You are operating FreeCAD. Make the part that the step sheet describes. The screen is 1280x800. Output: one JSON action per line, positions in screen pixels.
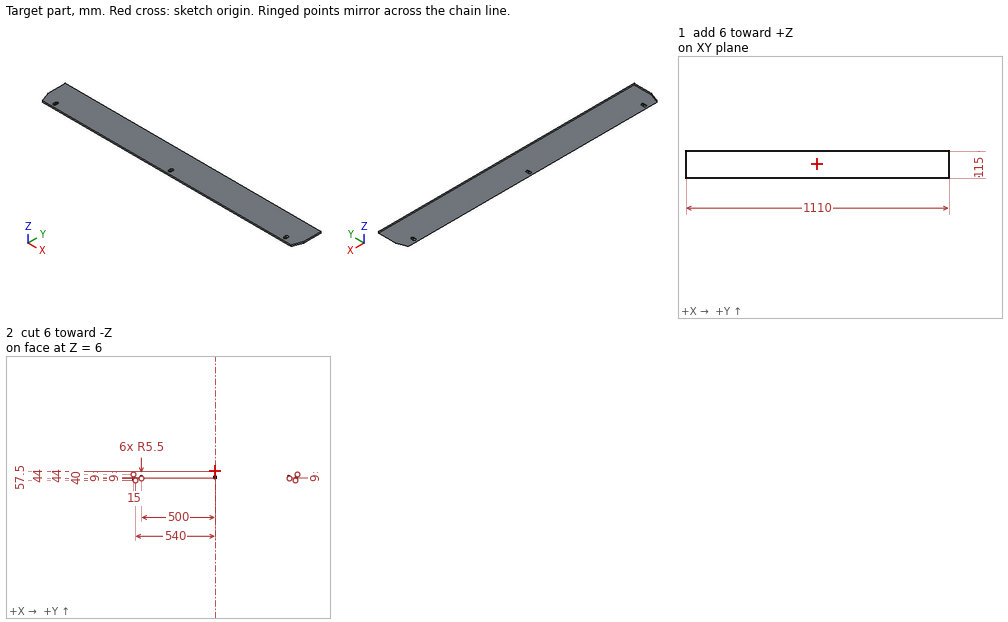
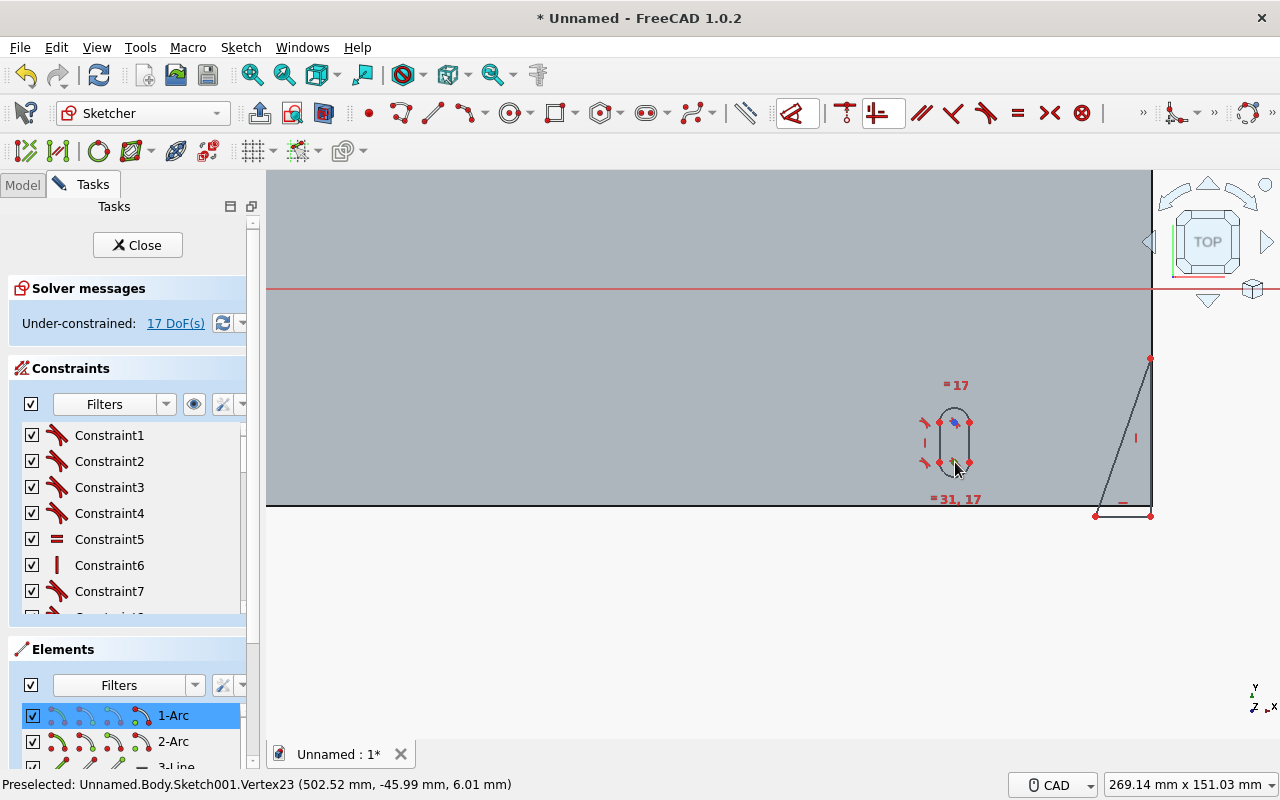
{"action": "scroll", "coordinate": [962, 463], "scroll_direction": "down", "scroll_amount": 10}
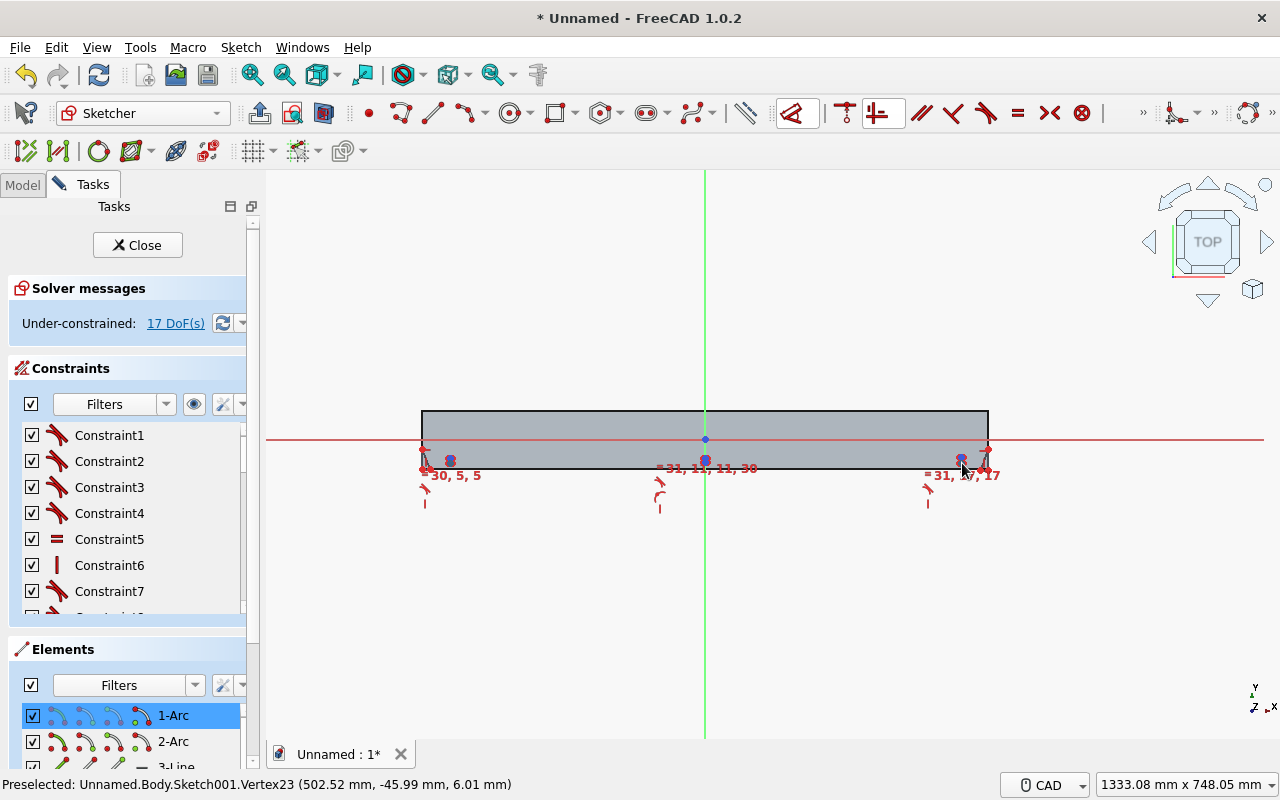
{"action": "left_click", "coordinate": [705, 674]}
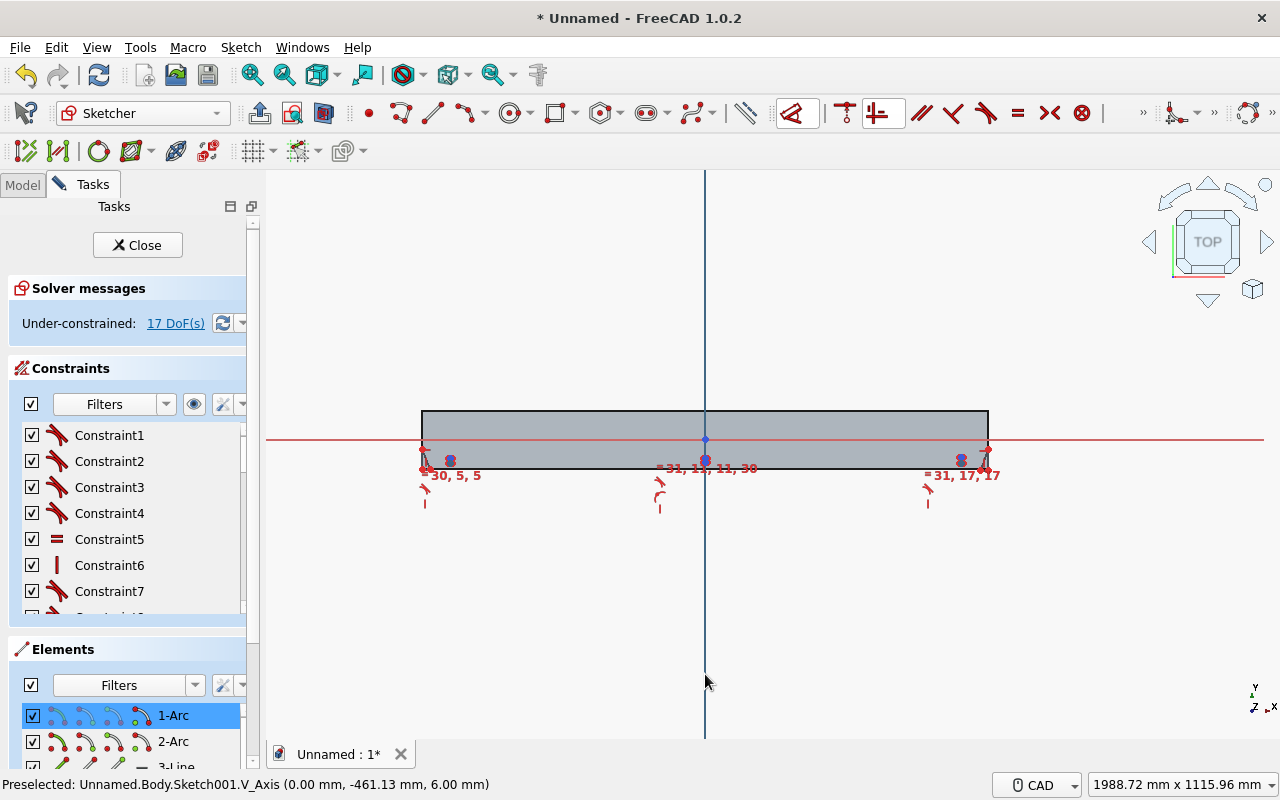
{"action": "left_click", "coordinate": [1050, 114]}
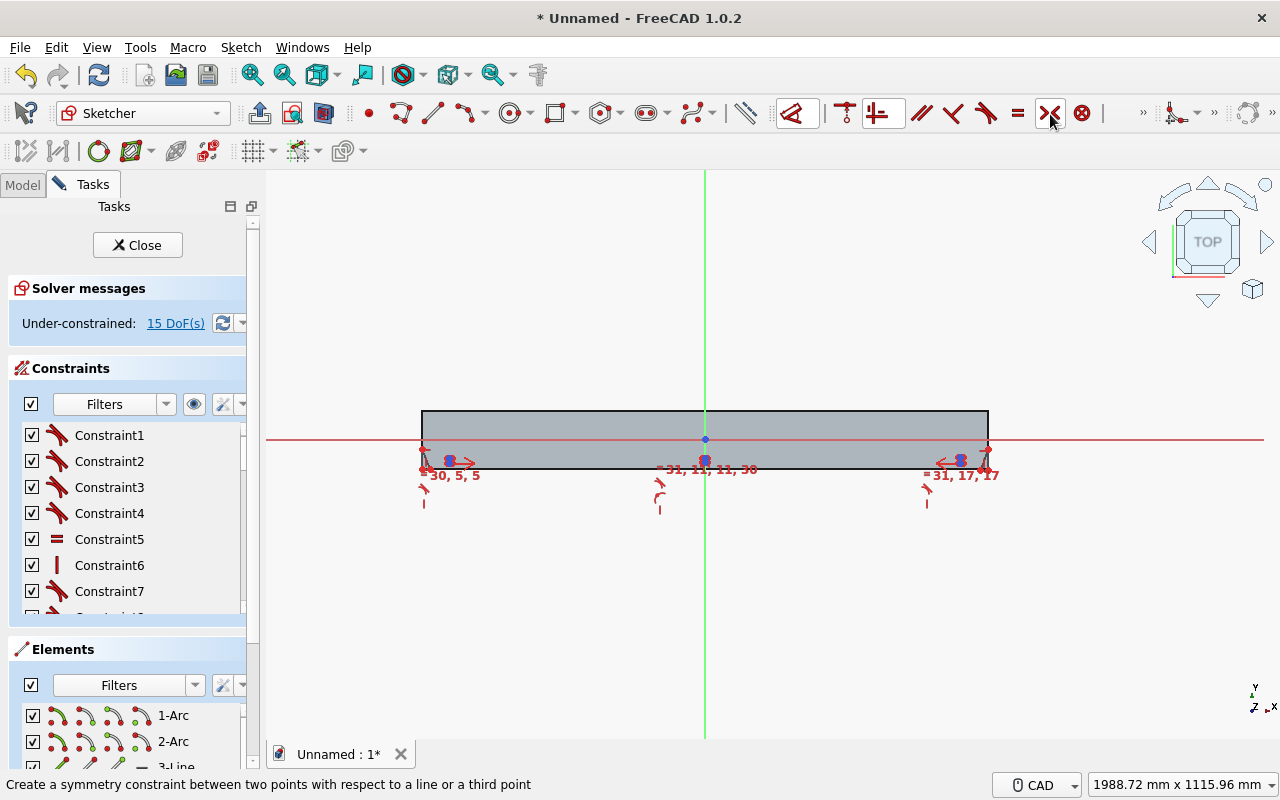
{"action": "scroll", "coordinate": [430, 470], "scroll_direction": "up", "scroll_amount": 3}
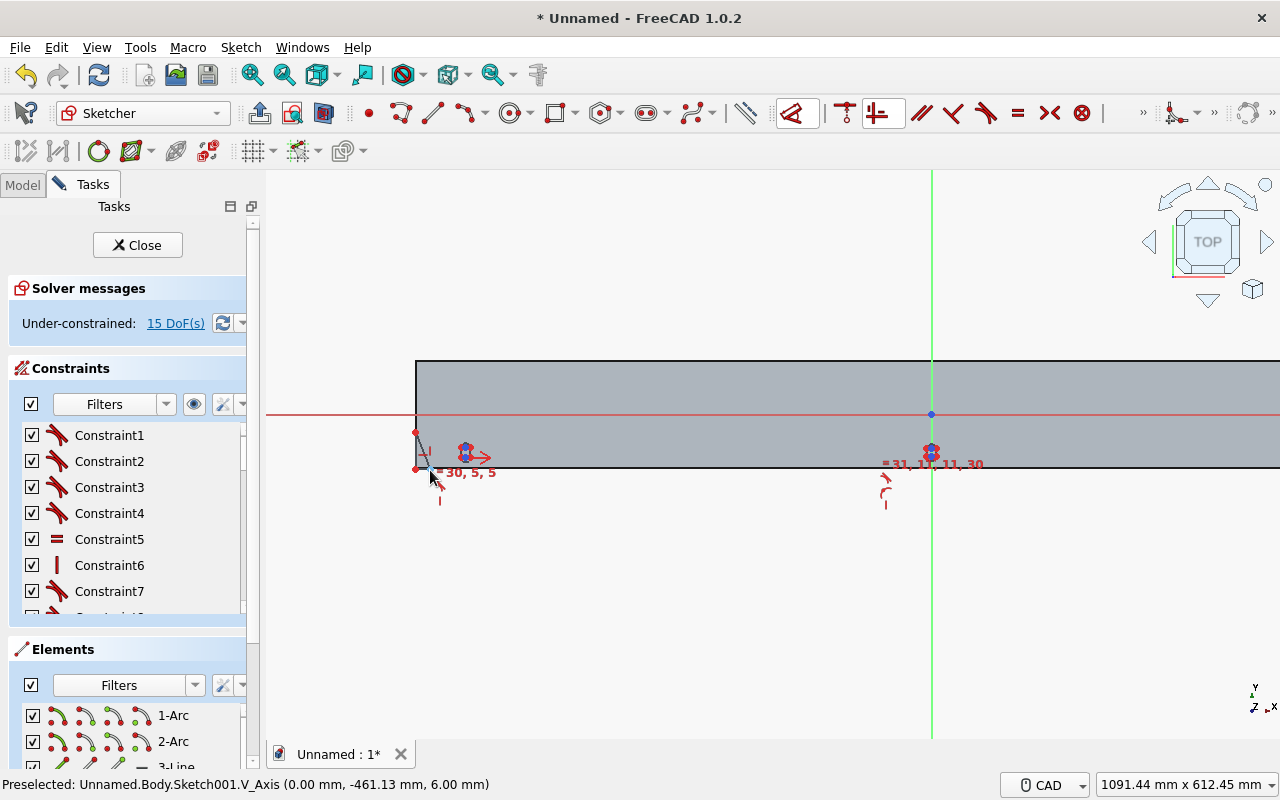
{"action": "left_click", "coordinate": [430, 469]}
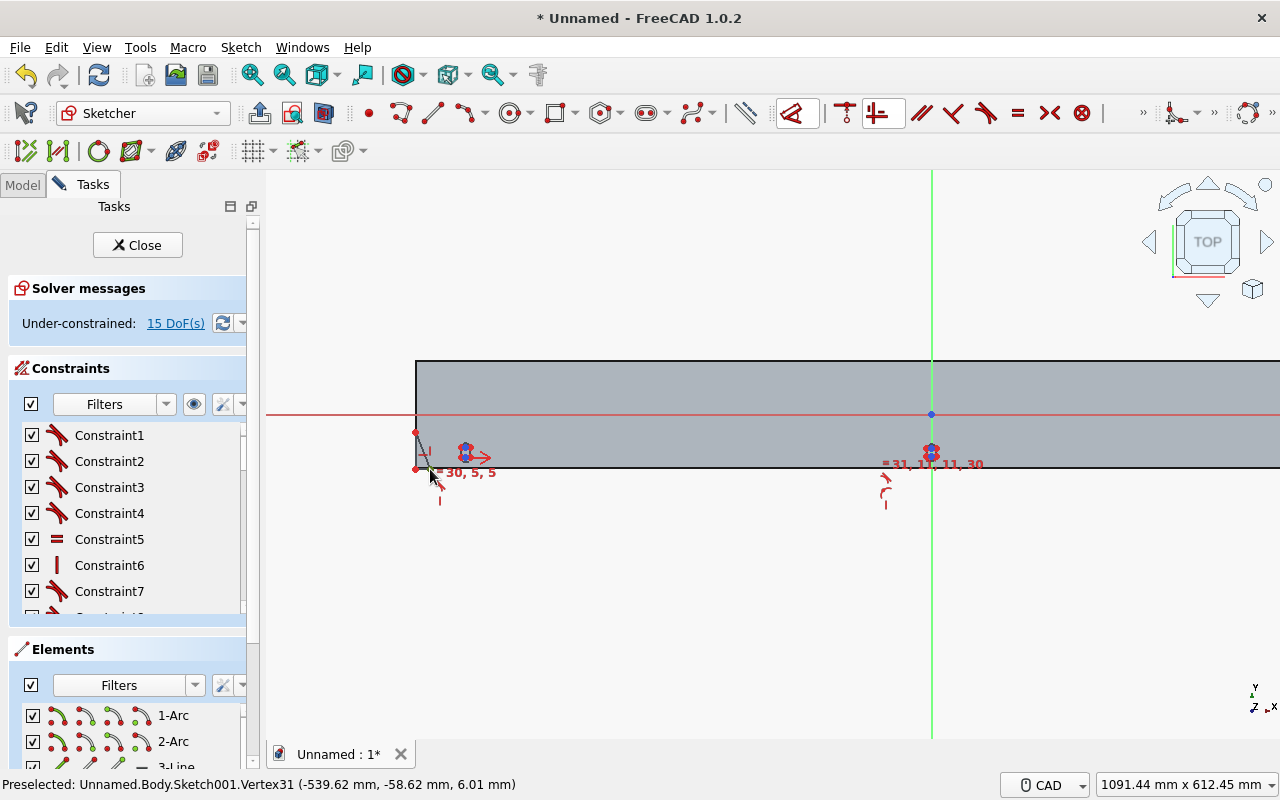
{"action": "scroll", "coordinate": [428, 470], "scroll_direction": "down", "scroll_amount": 3}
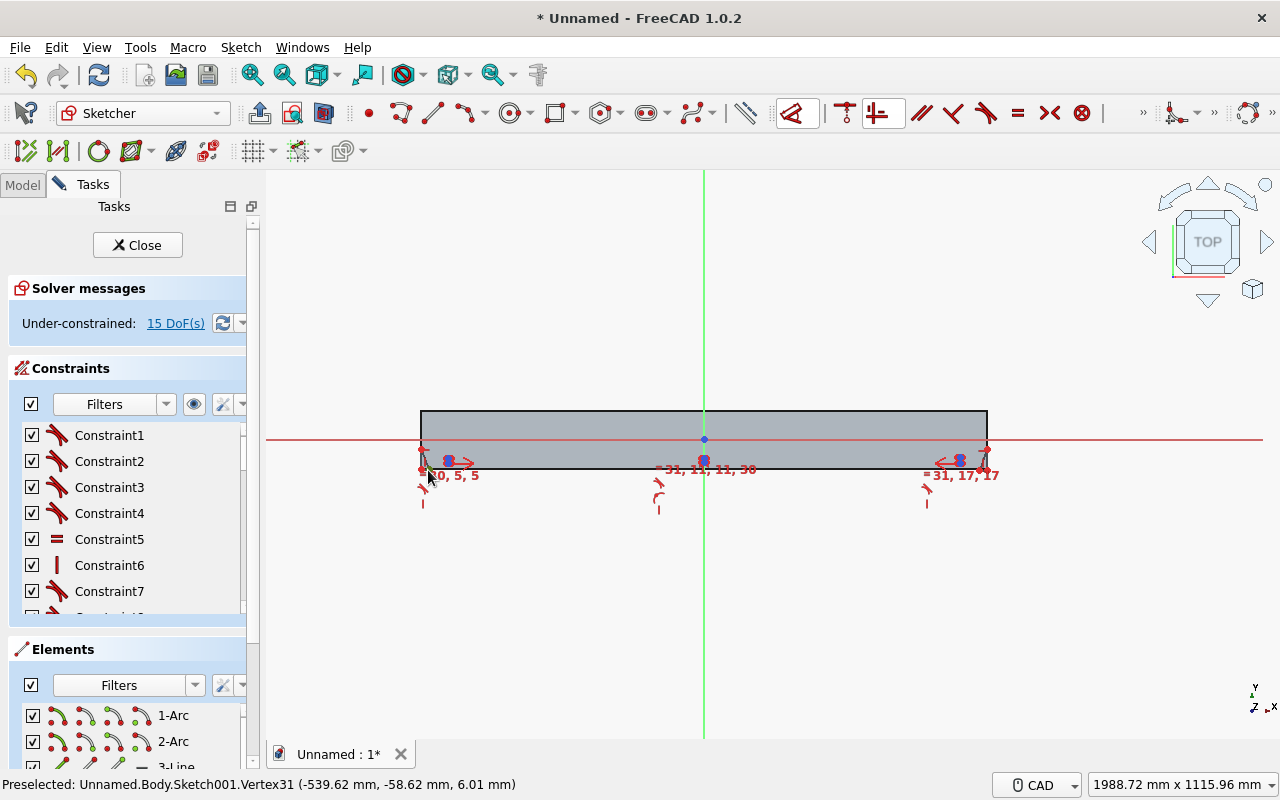
{"action": "scroll", "coordinate": [980, 471], "scroll_direction": "up", "scroll_amount": 3}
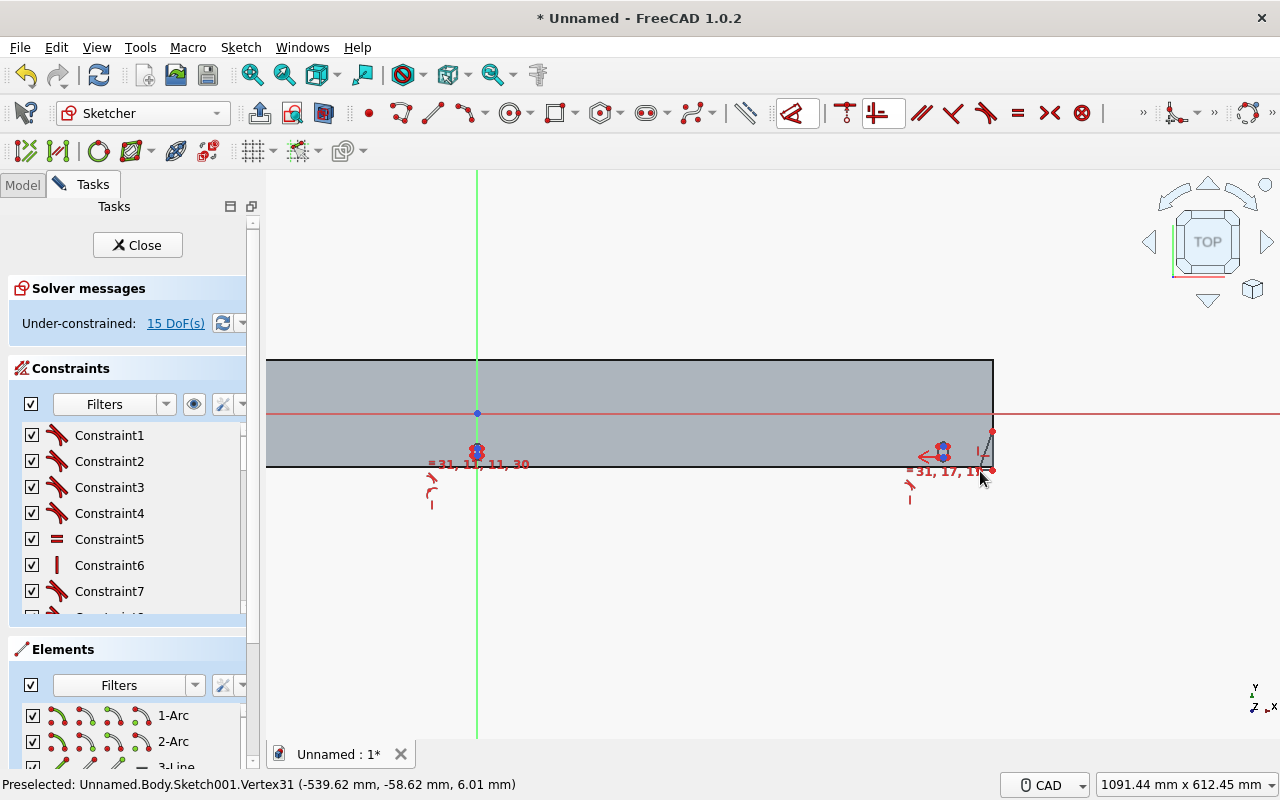
{"action": "scroll", "coordinate": [979, 470], "scroll_direction": "up", "scroll_amount": 4}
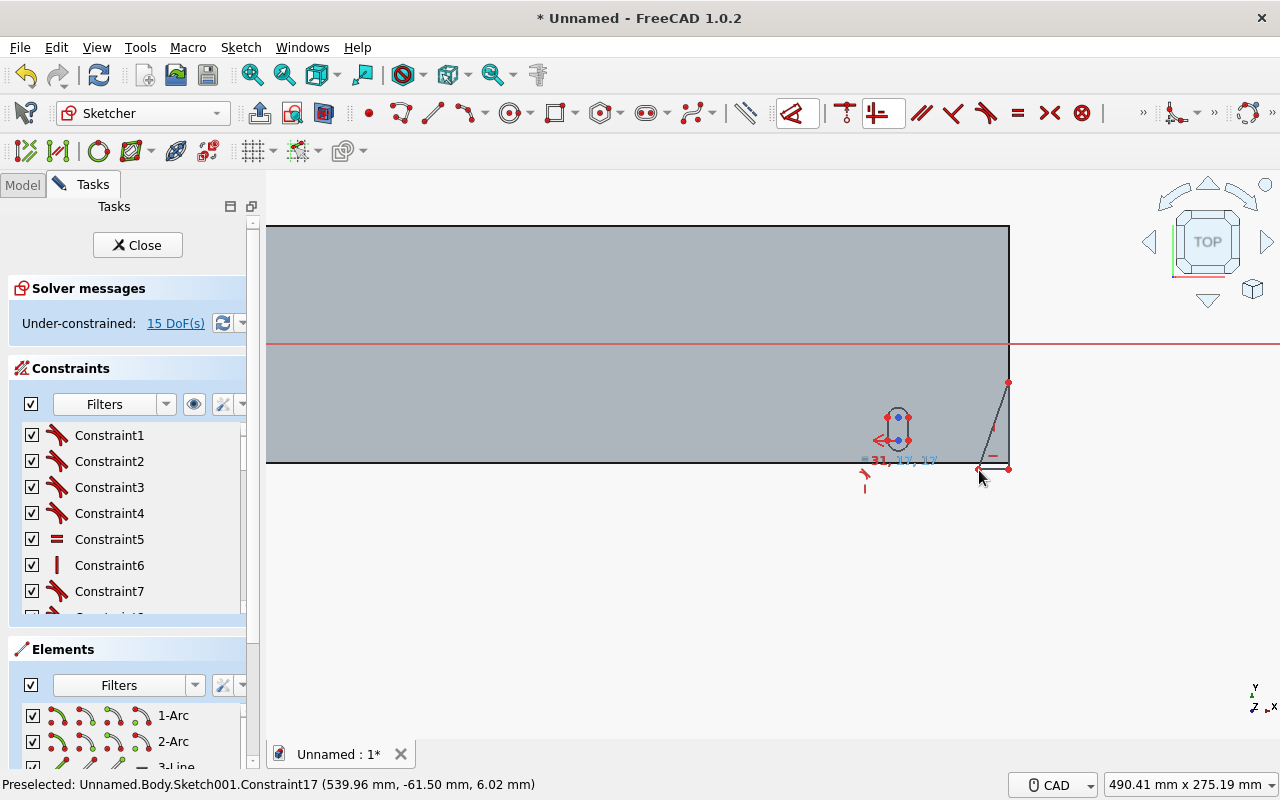
{"action": "left_click", "coordinate": [978, 469]}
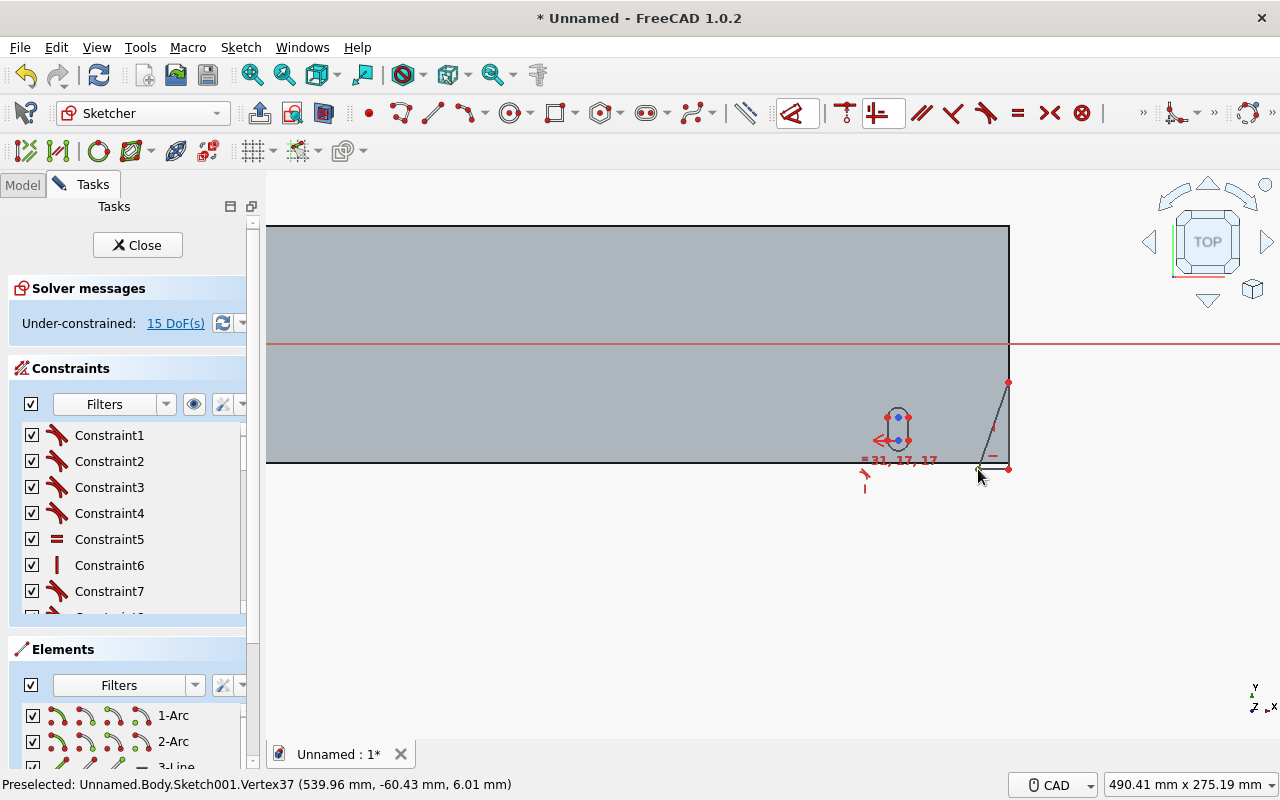
{"action": "scroll", "coordinate": [980, 471], "scroll_direction": "down", "scroll_amount": 7}